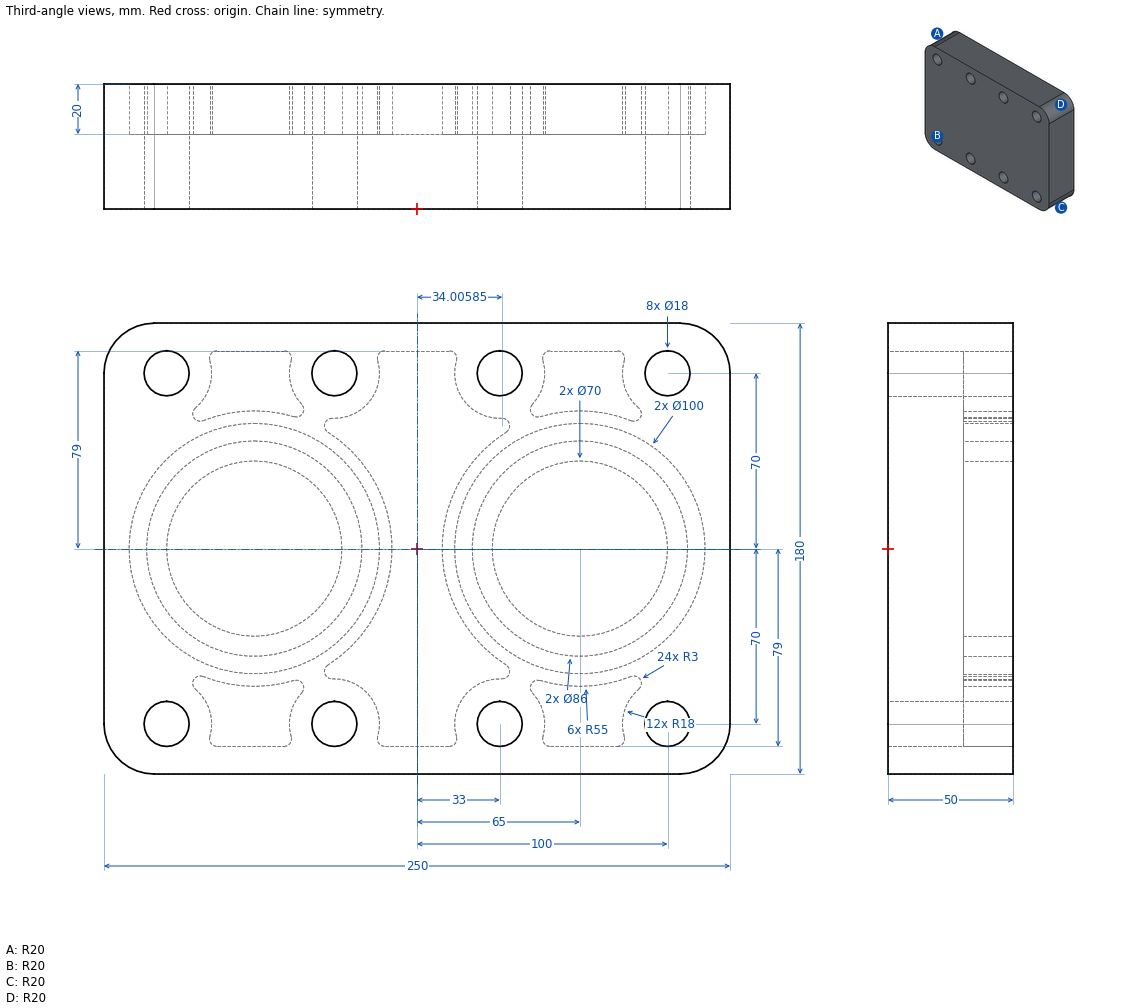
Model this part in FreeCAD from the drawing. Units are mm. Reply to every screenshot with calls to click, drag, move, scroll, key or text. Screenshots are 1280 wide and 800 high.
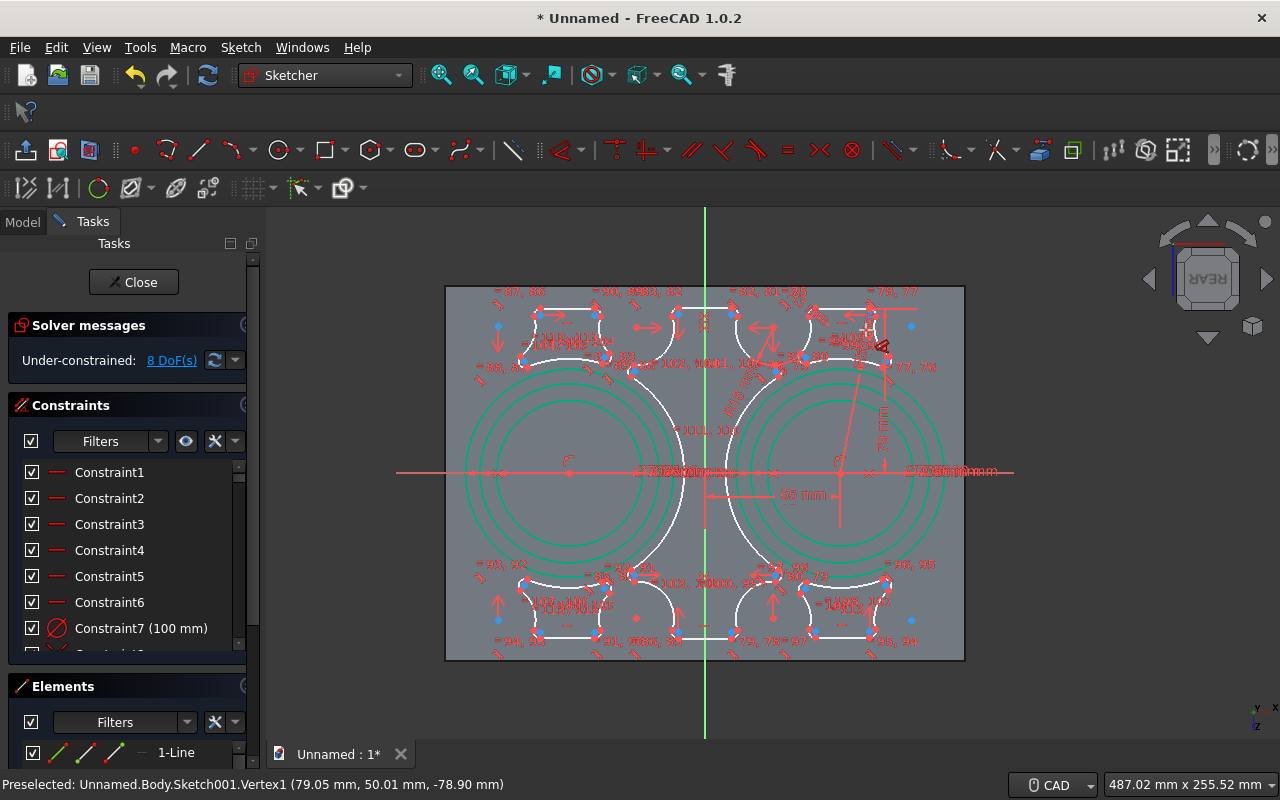
scroll(678, 639, up, 4)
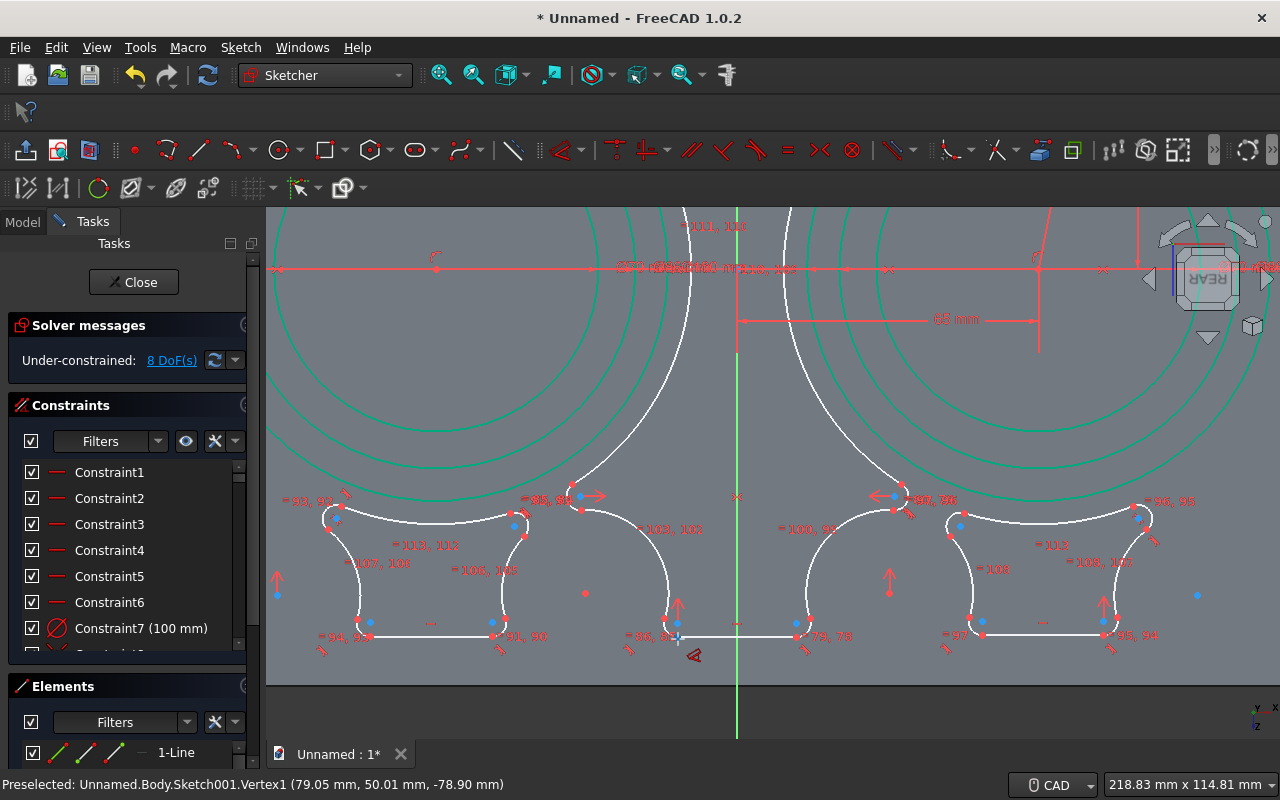
click(678, 637)
click(644, 453)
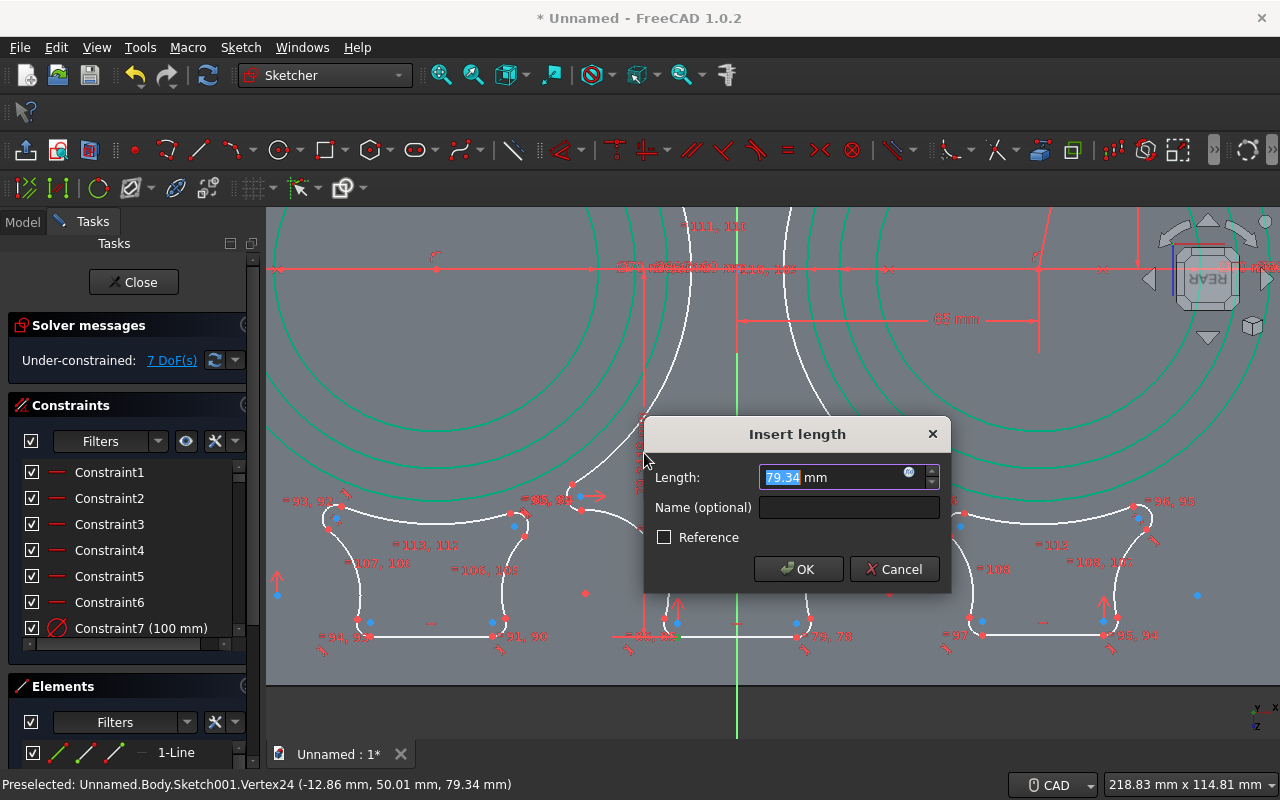
text(79)
key(Return)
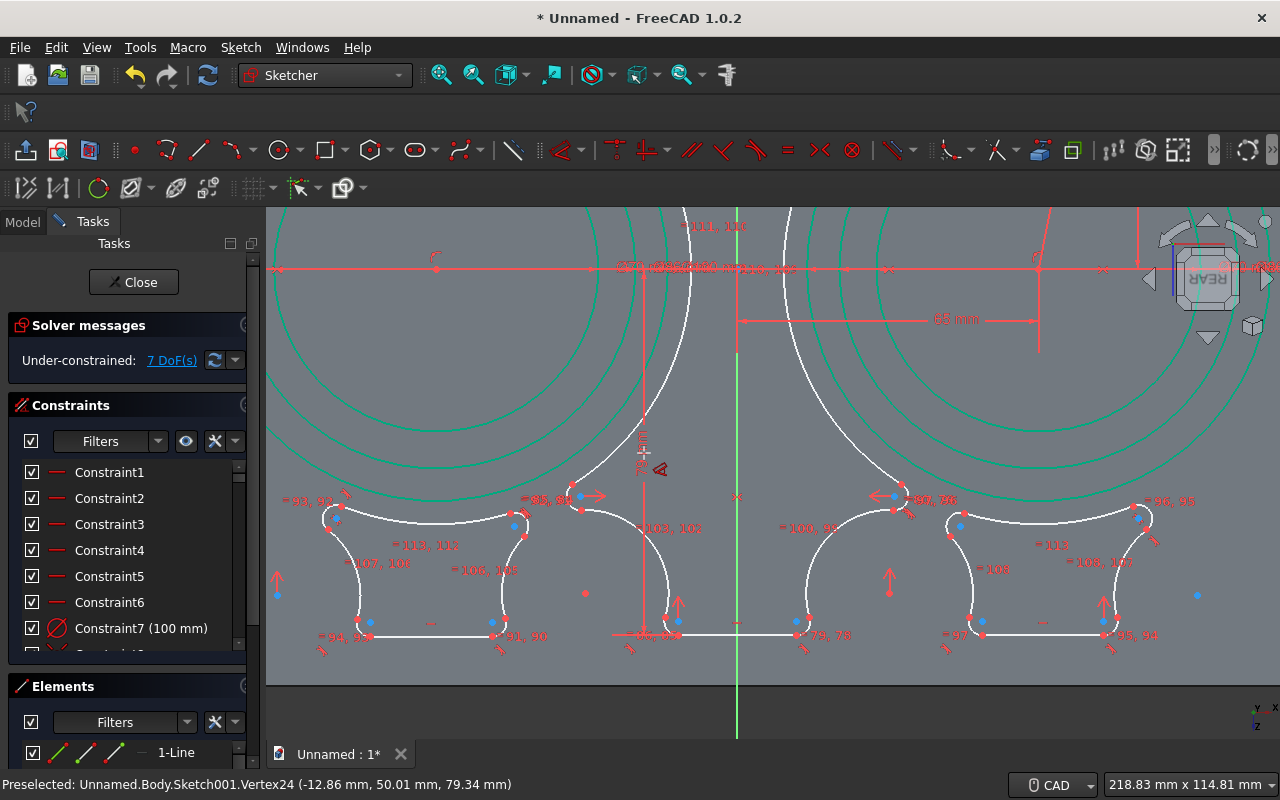
click(371, 637)
click(337, 369)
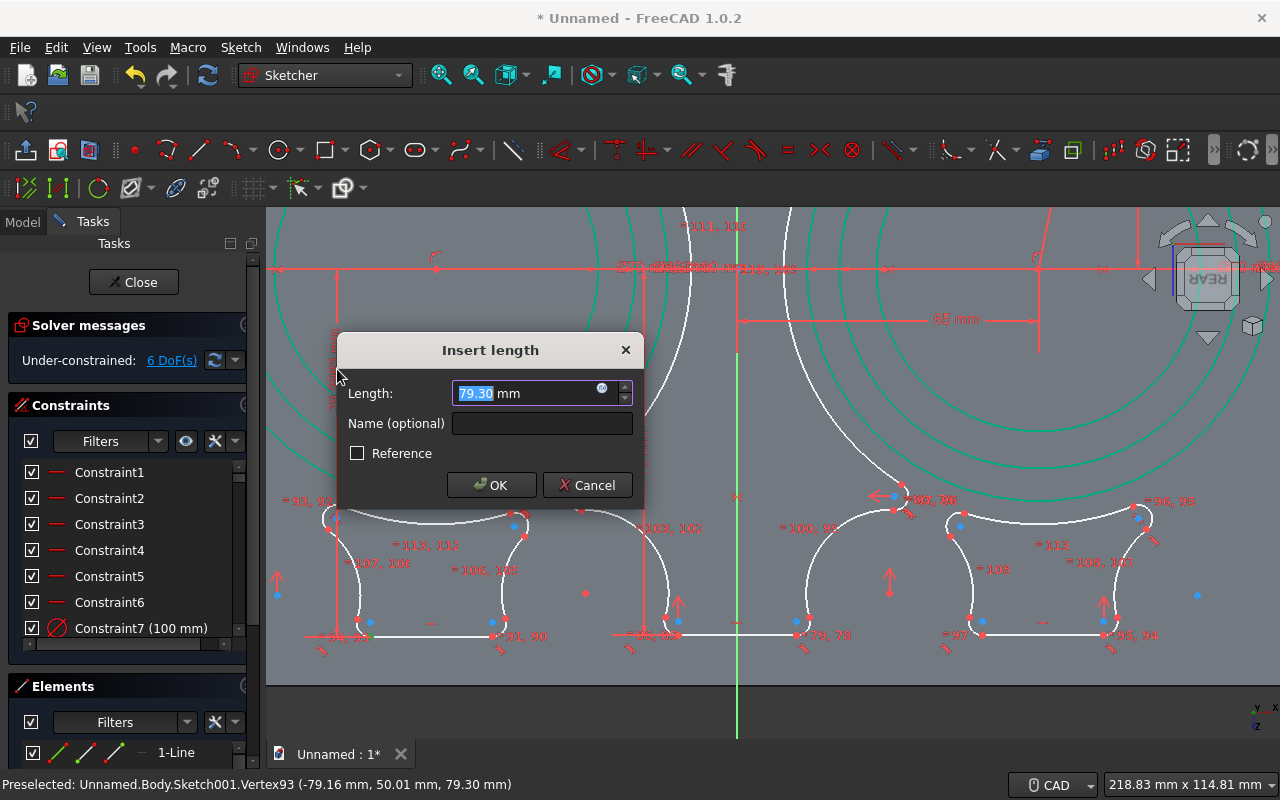
text(79)
key(Return)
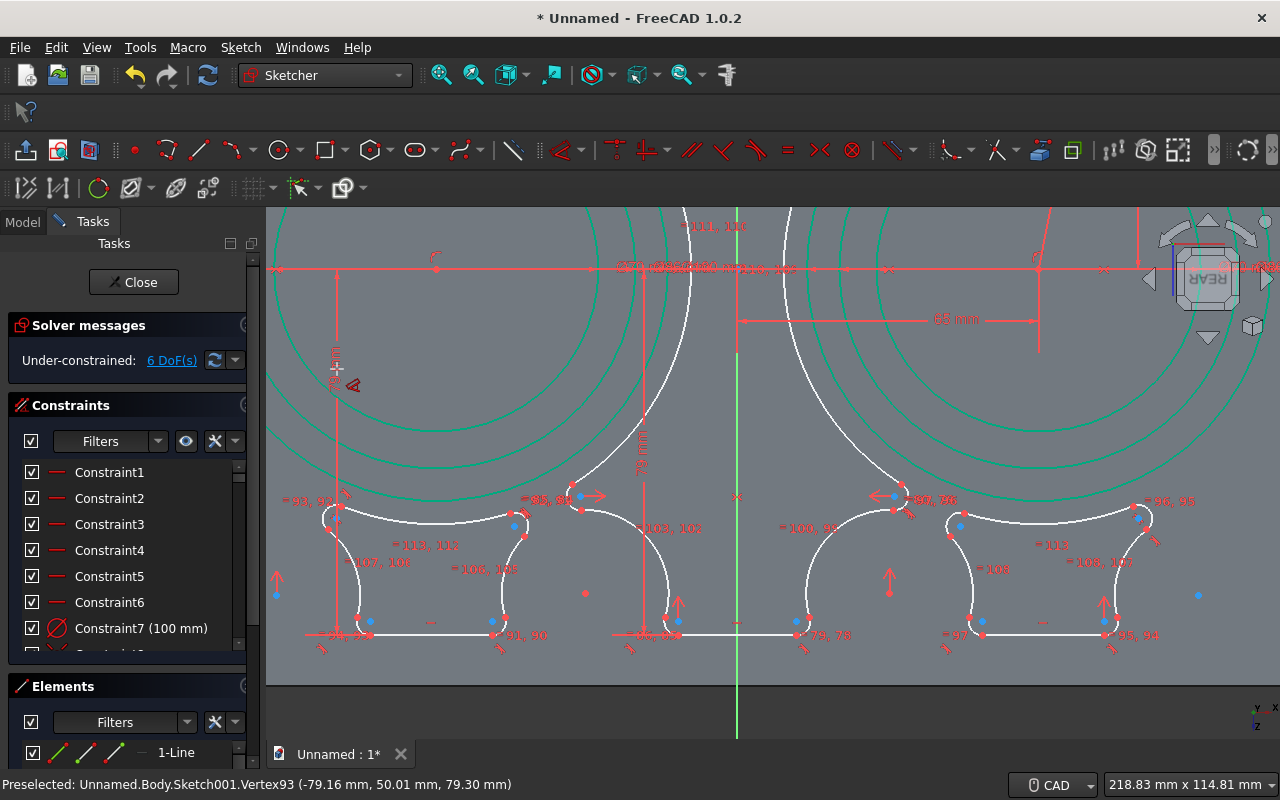
scroll(678, 639, down, 4)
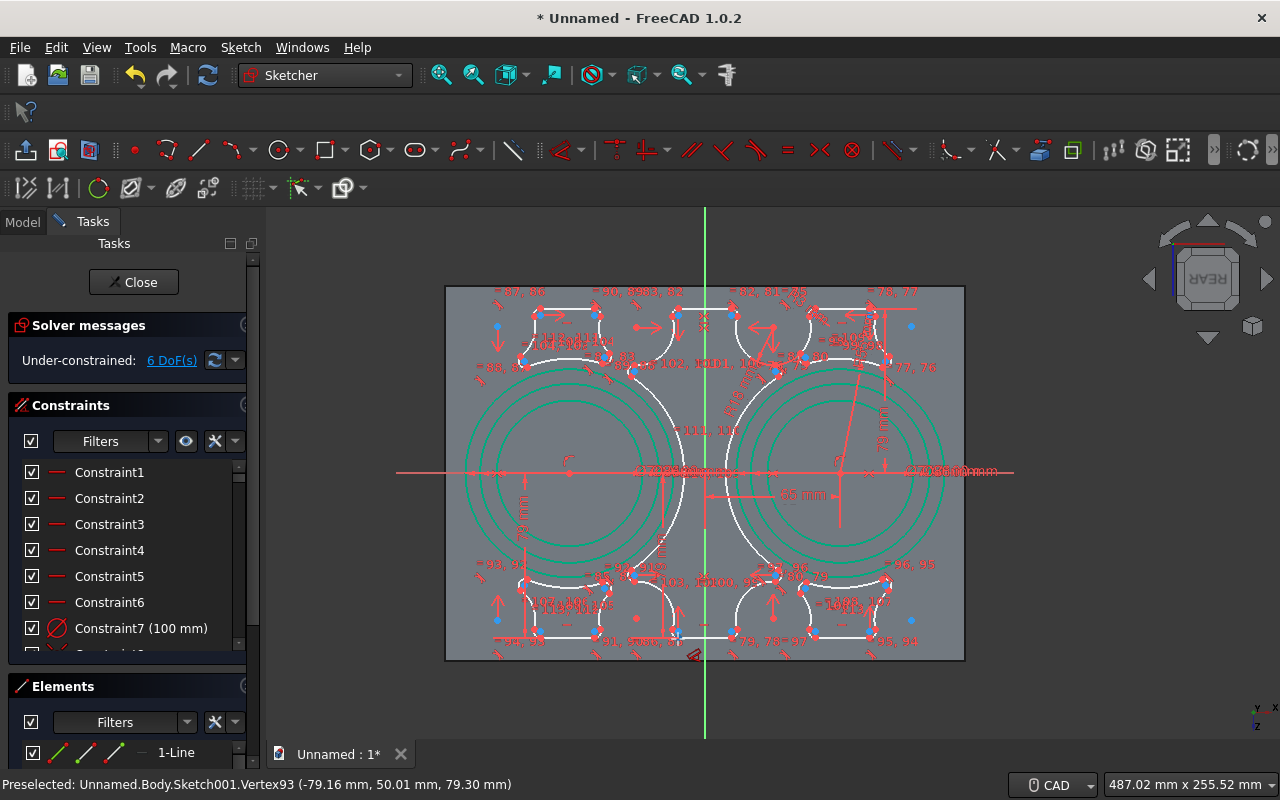
click(773, 328)
click(723, 294)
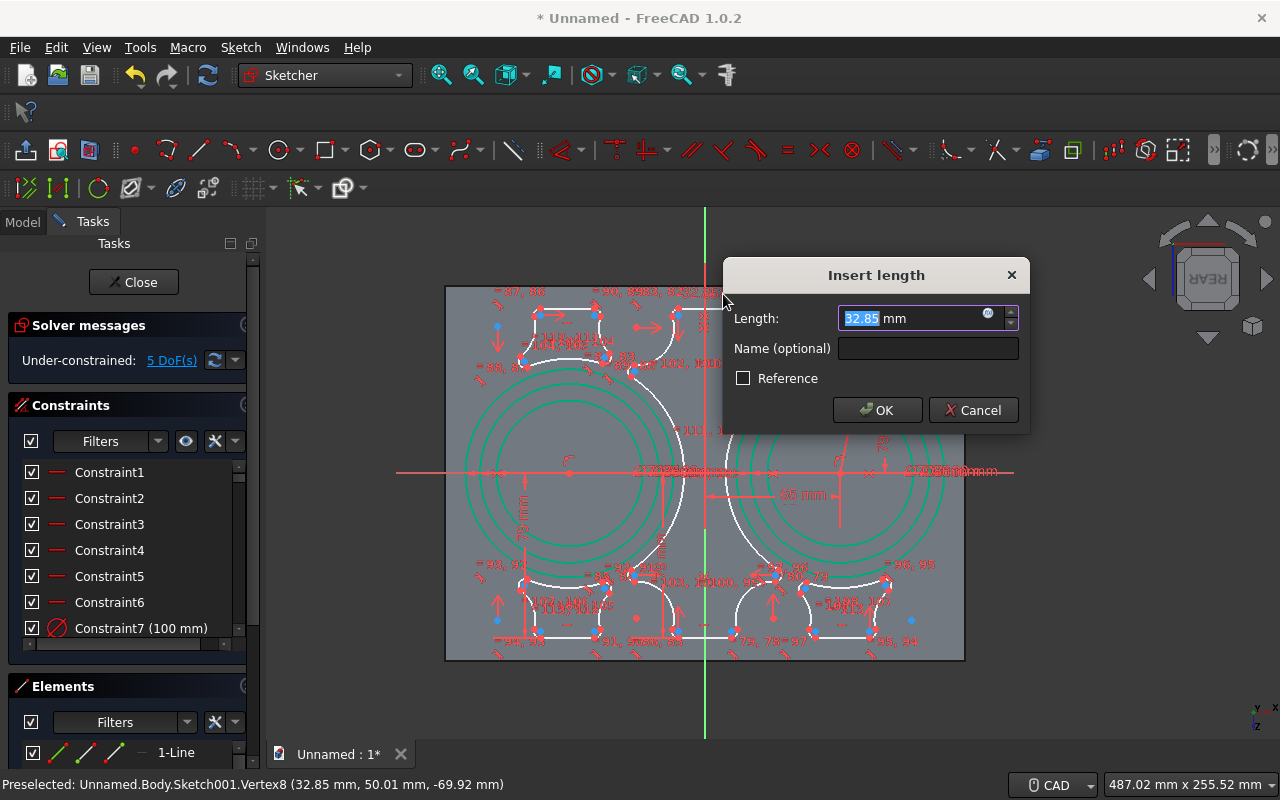
text(33)
key(Return)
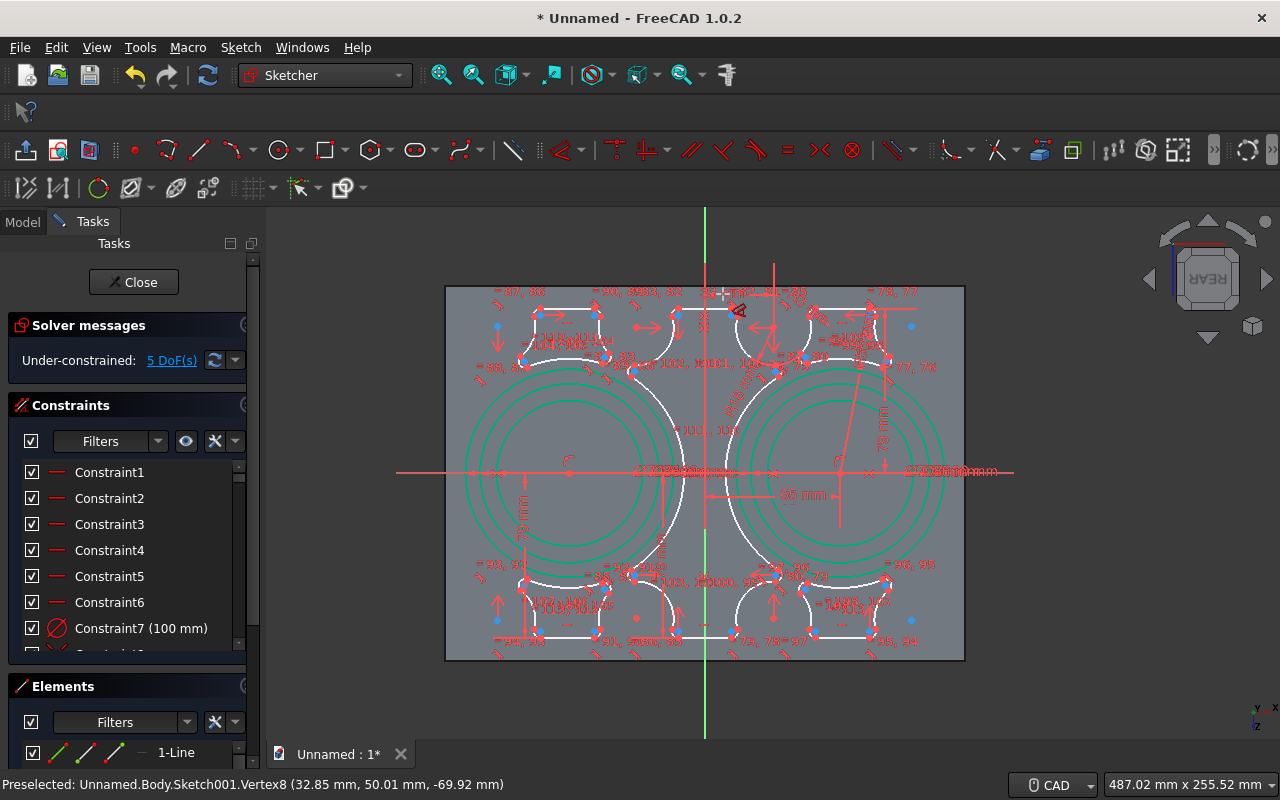
click(912, 327)
click(946, 400)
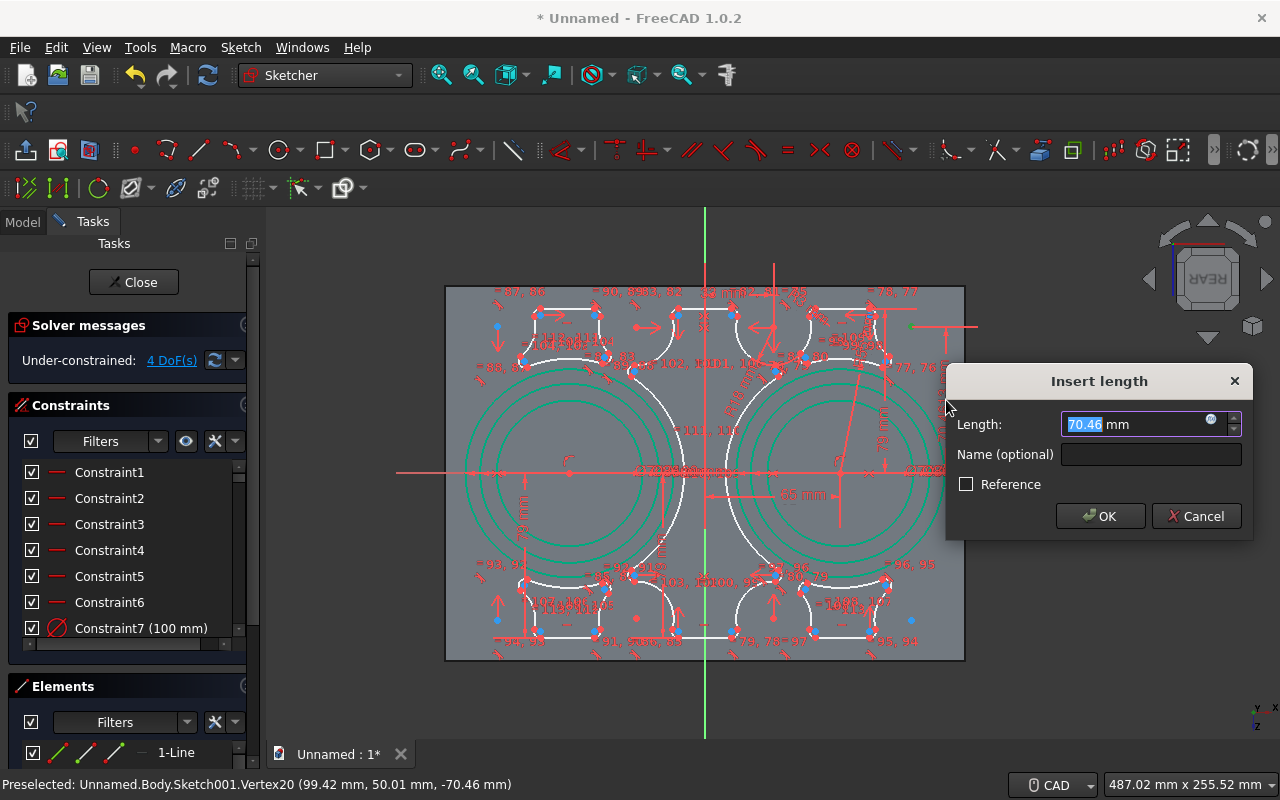
text(70)
key(Return)